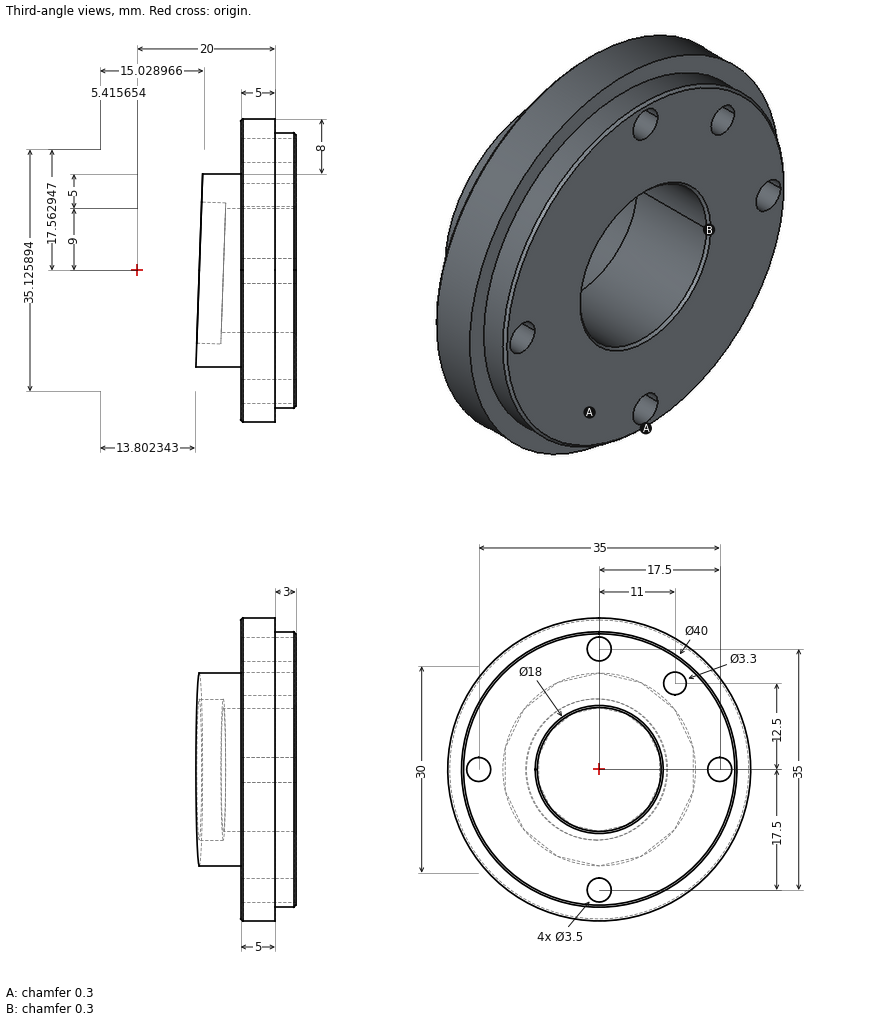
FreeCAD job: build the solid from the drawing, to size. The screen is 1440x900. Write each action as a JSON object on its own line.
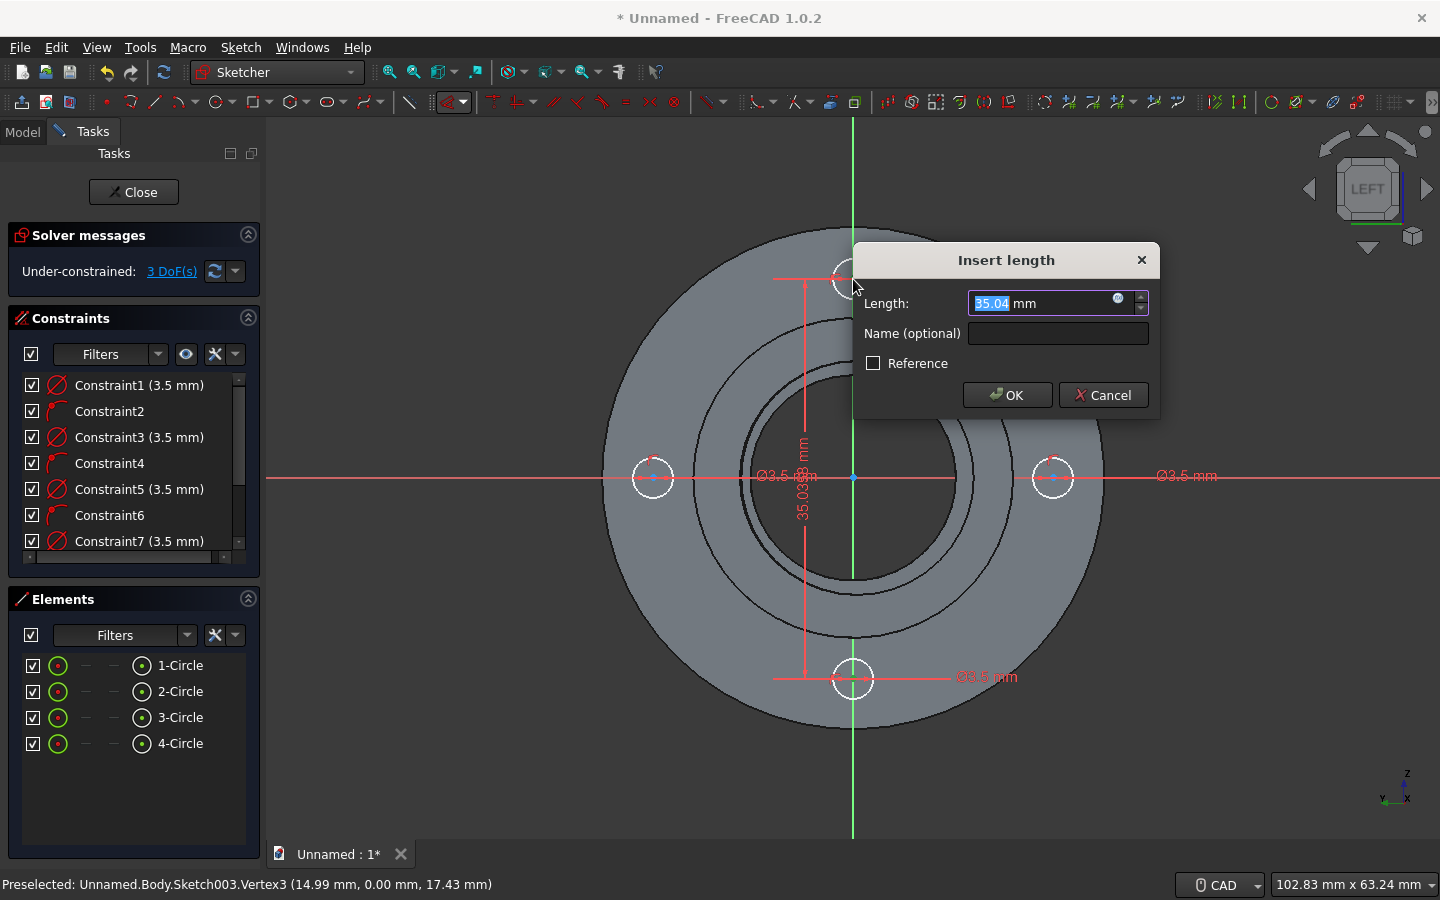
{"action": "type", "text": "35"}
{"action": "key", "text": "Return"}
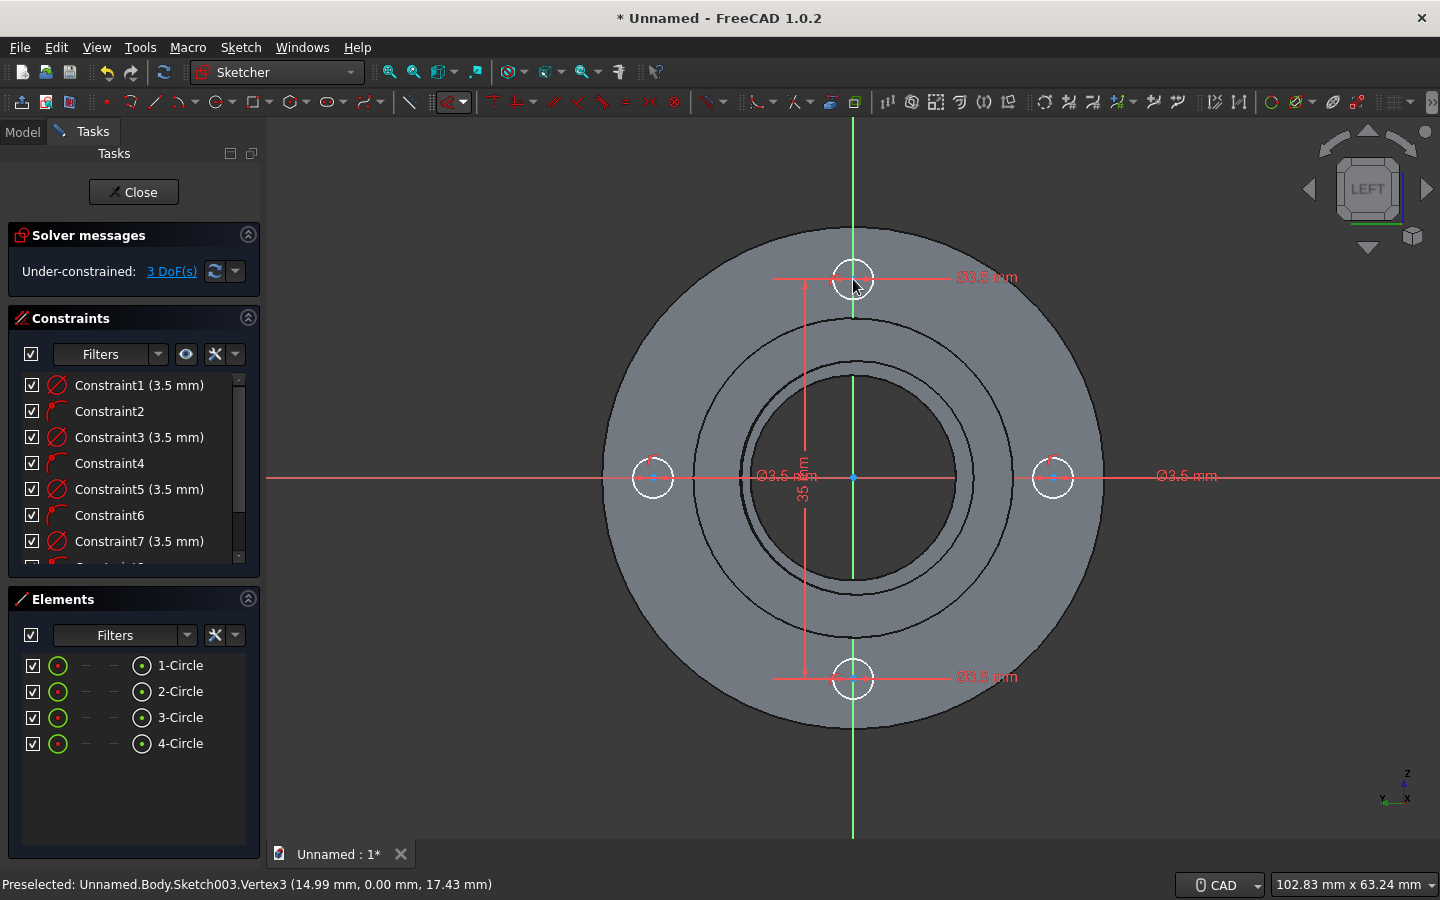
{"action": "left_click", "coordinate": [653, 478]}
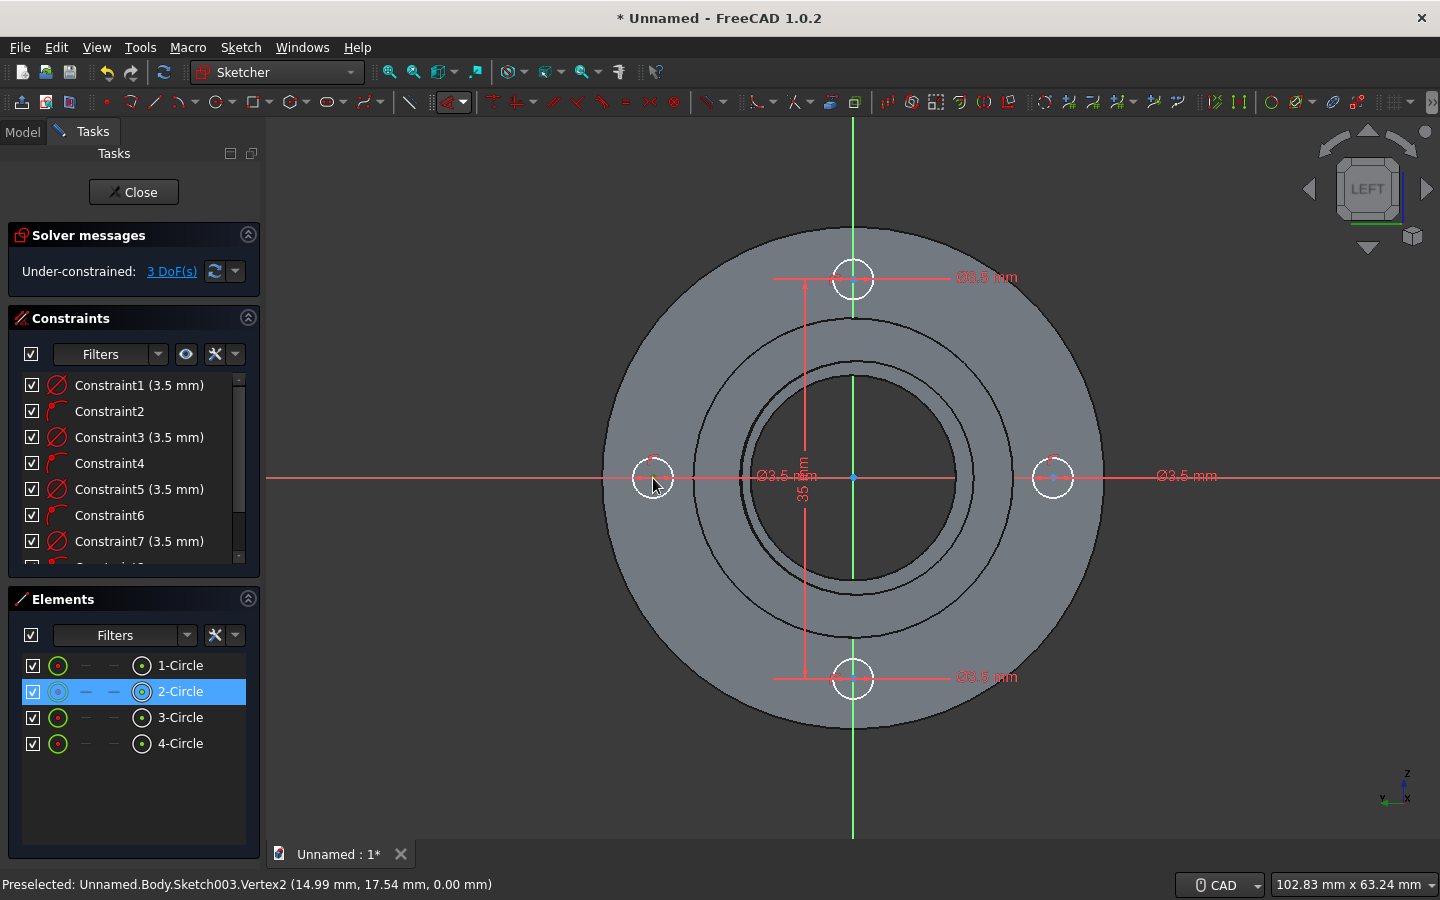
{"action": "left_click", "coordinate": [1053, 478]}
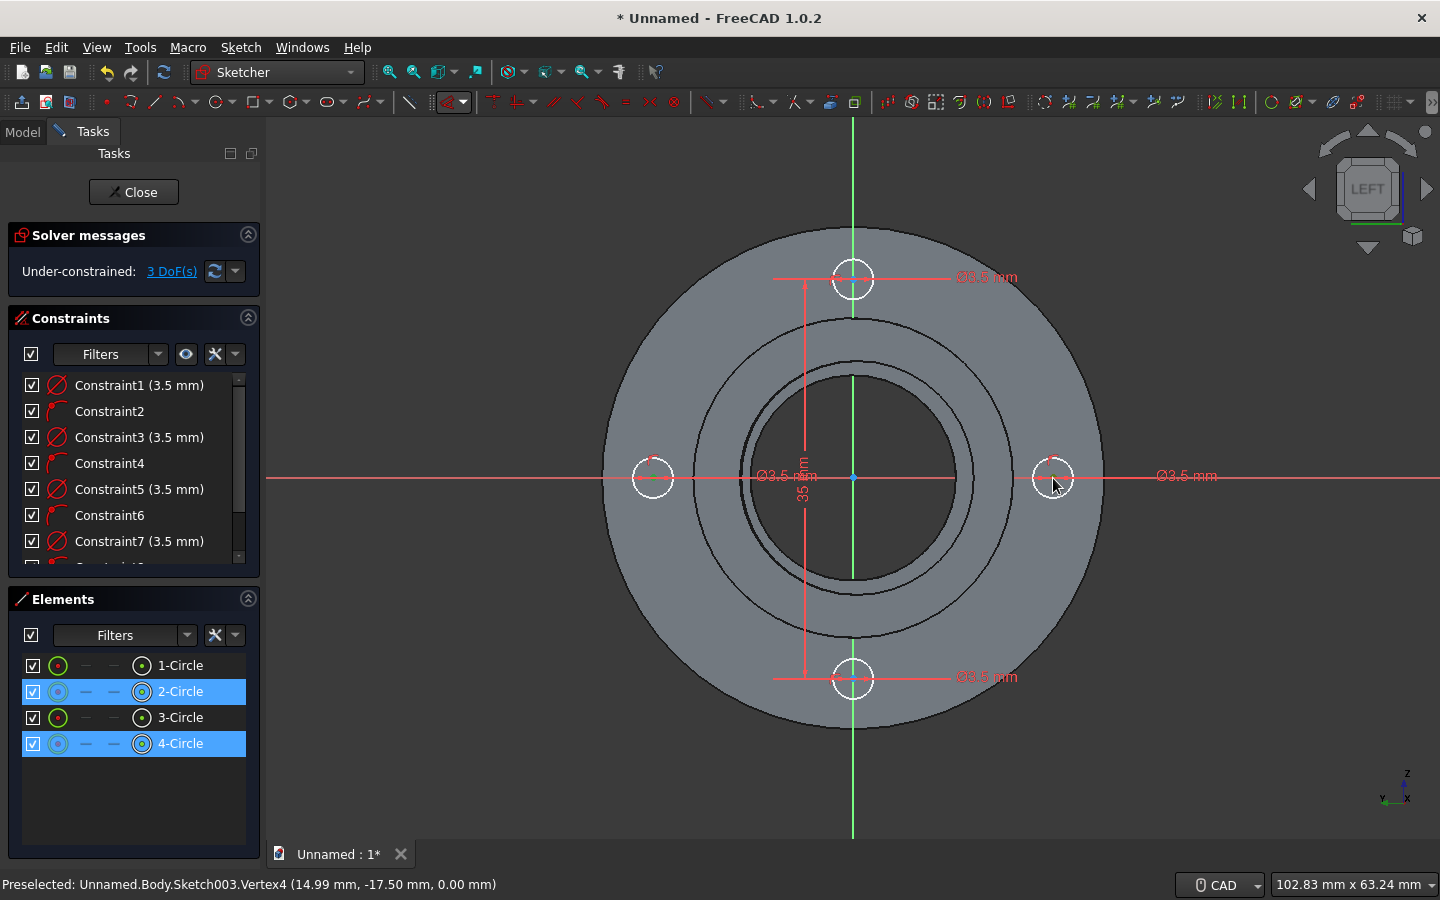
{"action": "key", "text": "l"}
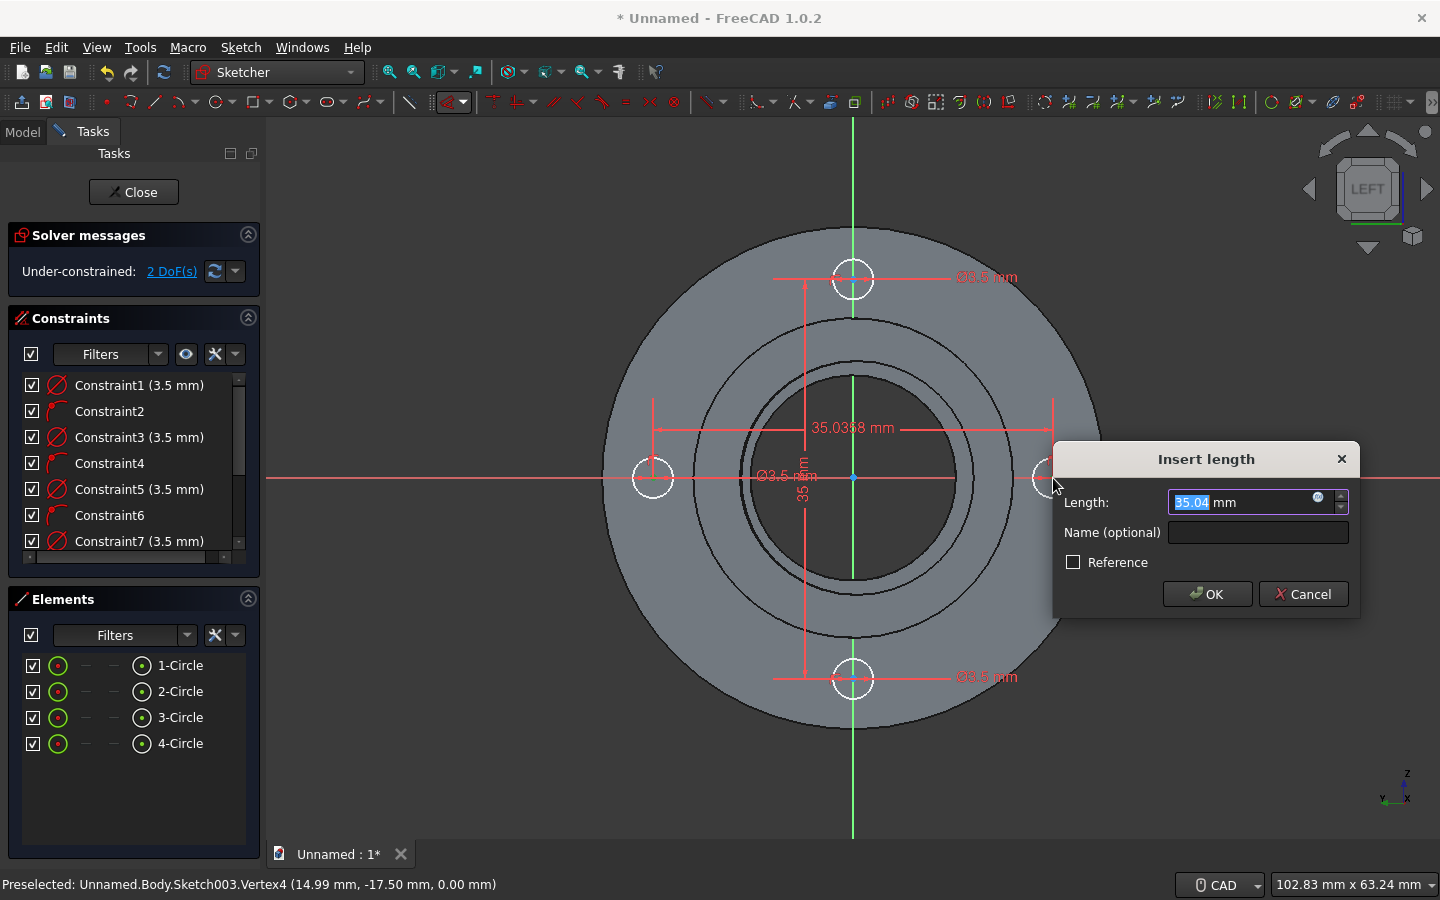
{"action": "type", "text": "35"}
{"action": "key", "text": "Return"}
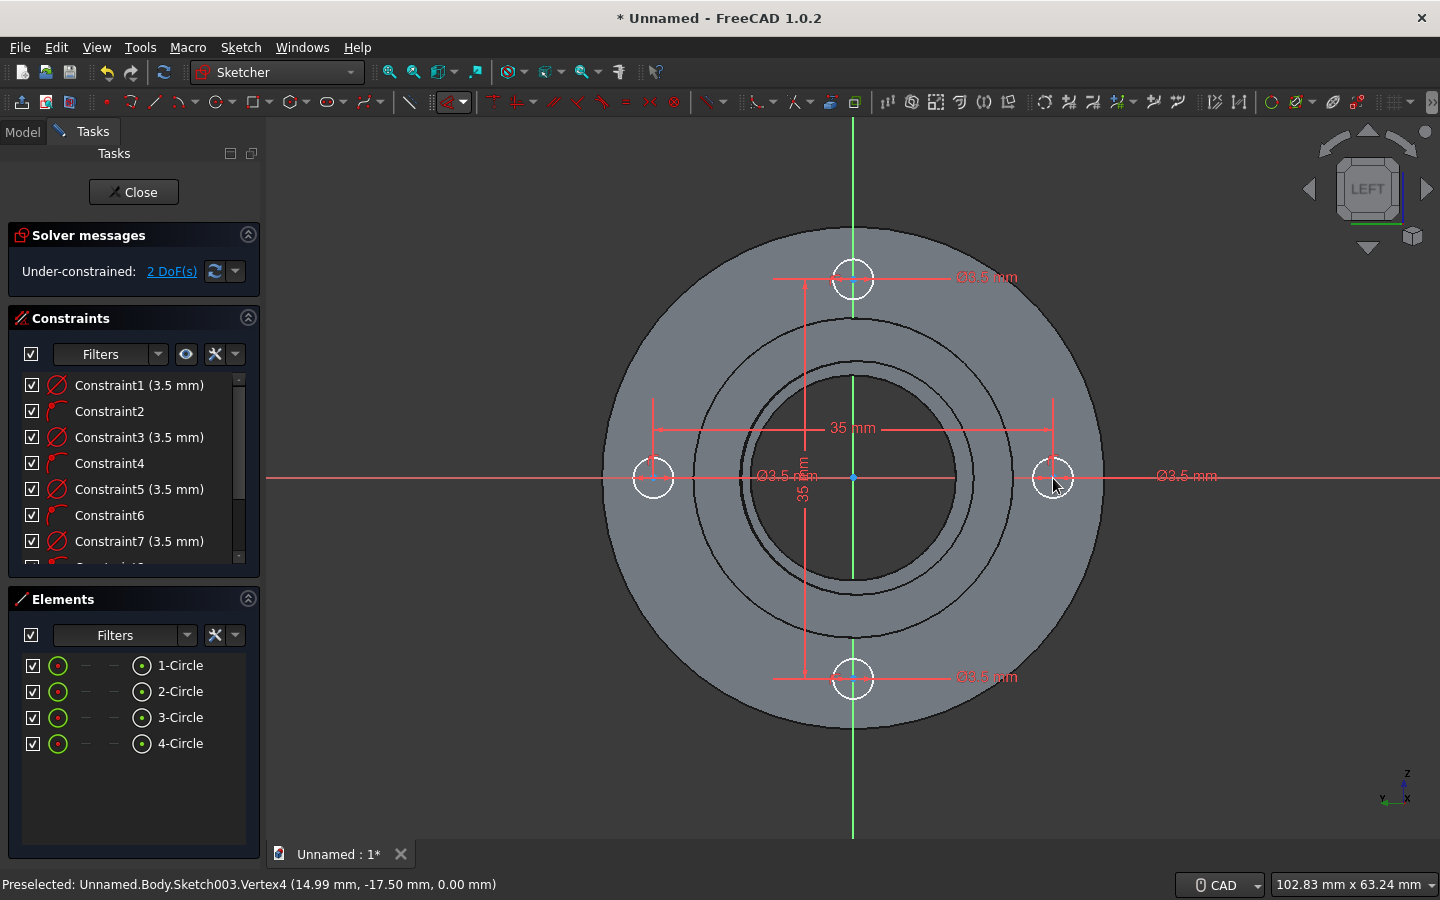
{"action": "left_click", "coordinate": [853, 679]}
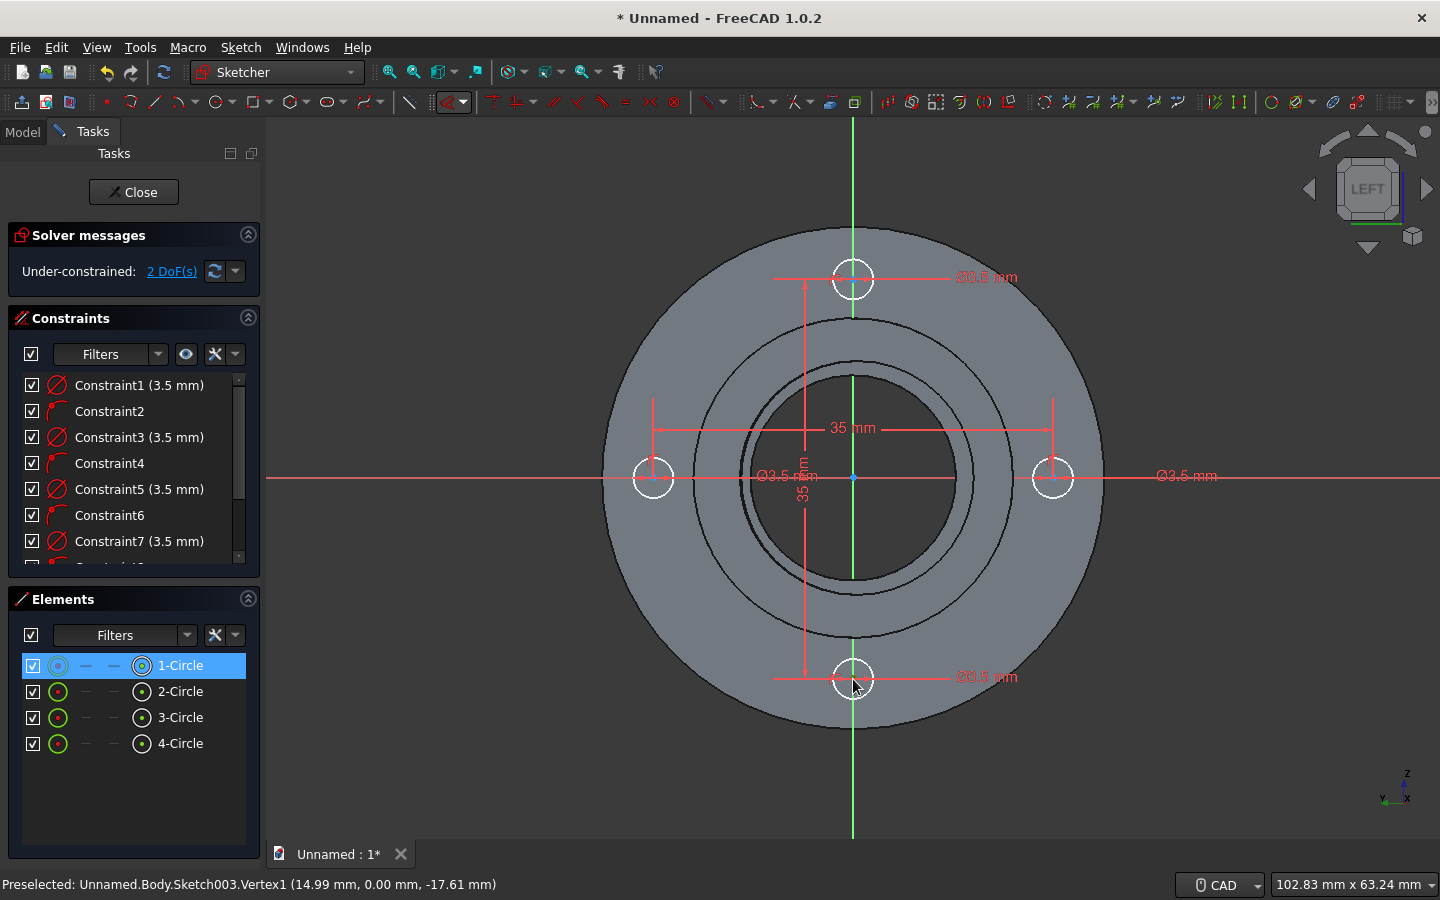
{"action": "left_click", "coordinate": [466, 102]}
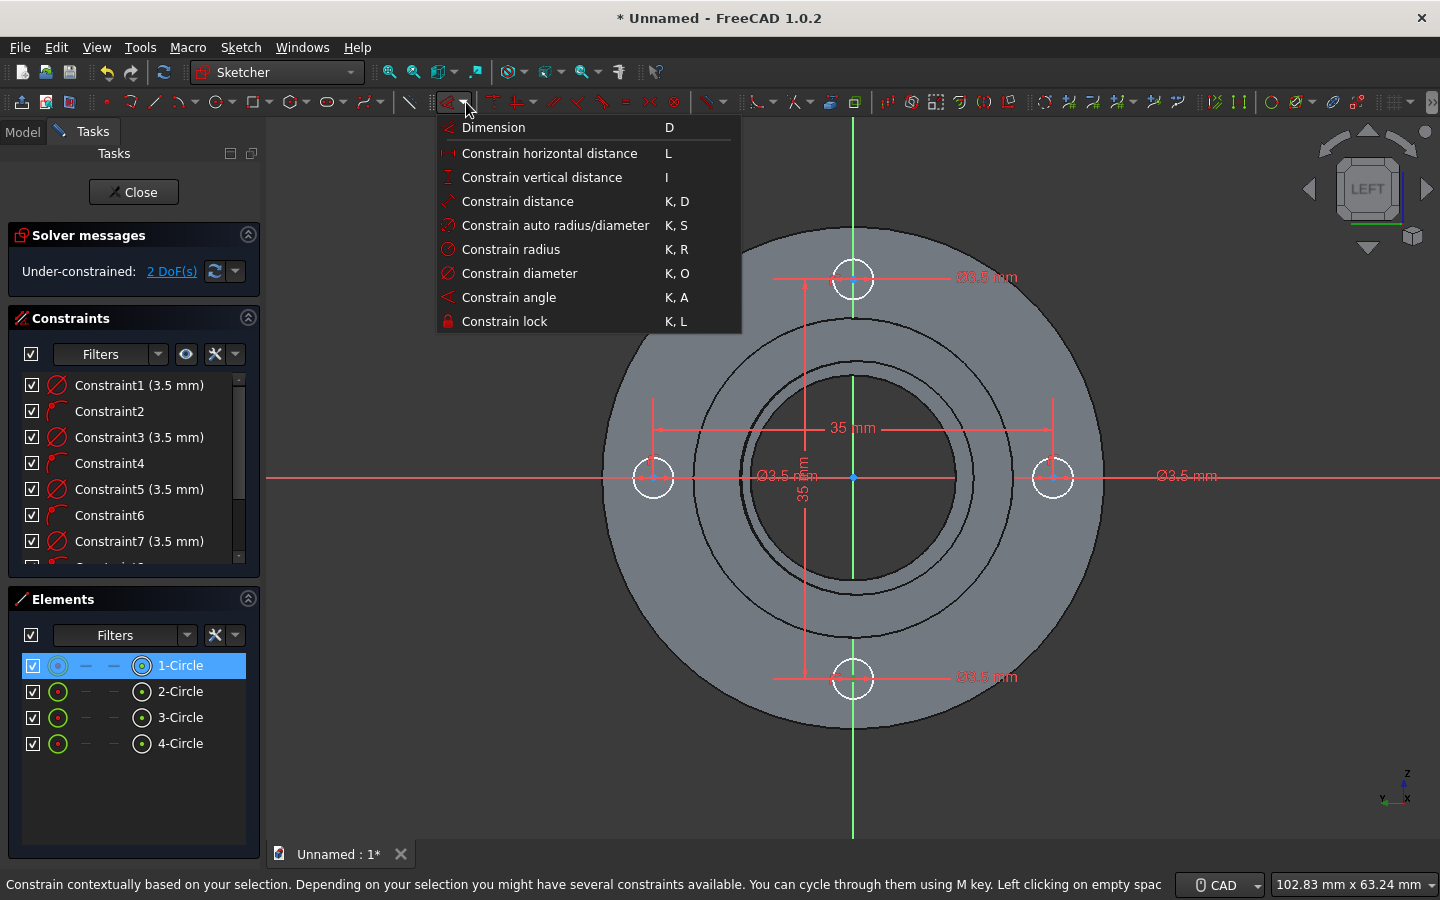
{"action": "left_click", "coordinate": [589, 177]}